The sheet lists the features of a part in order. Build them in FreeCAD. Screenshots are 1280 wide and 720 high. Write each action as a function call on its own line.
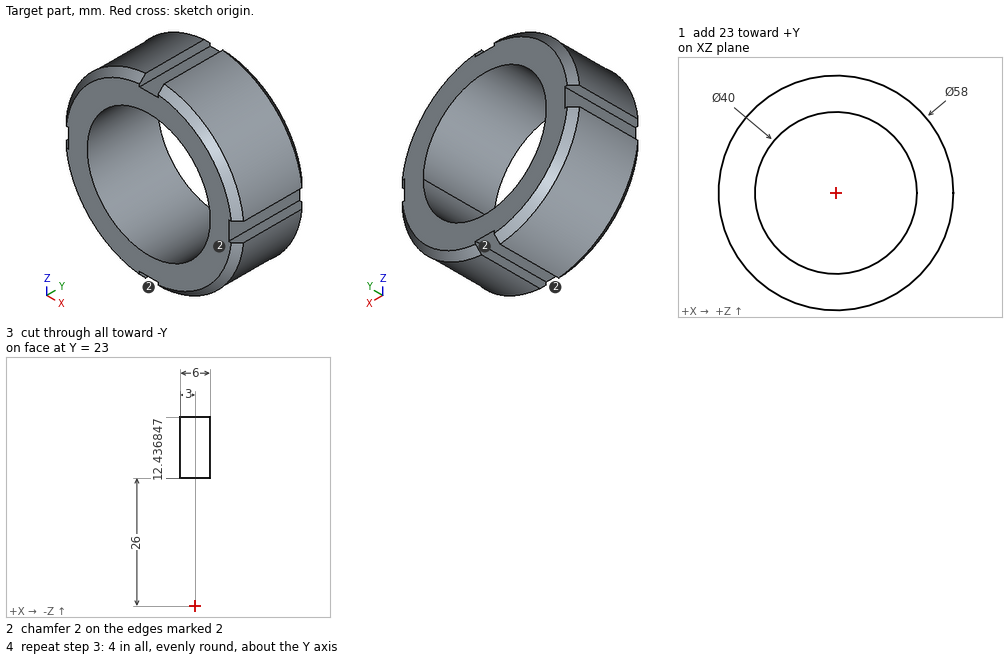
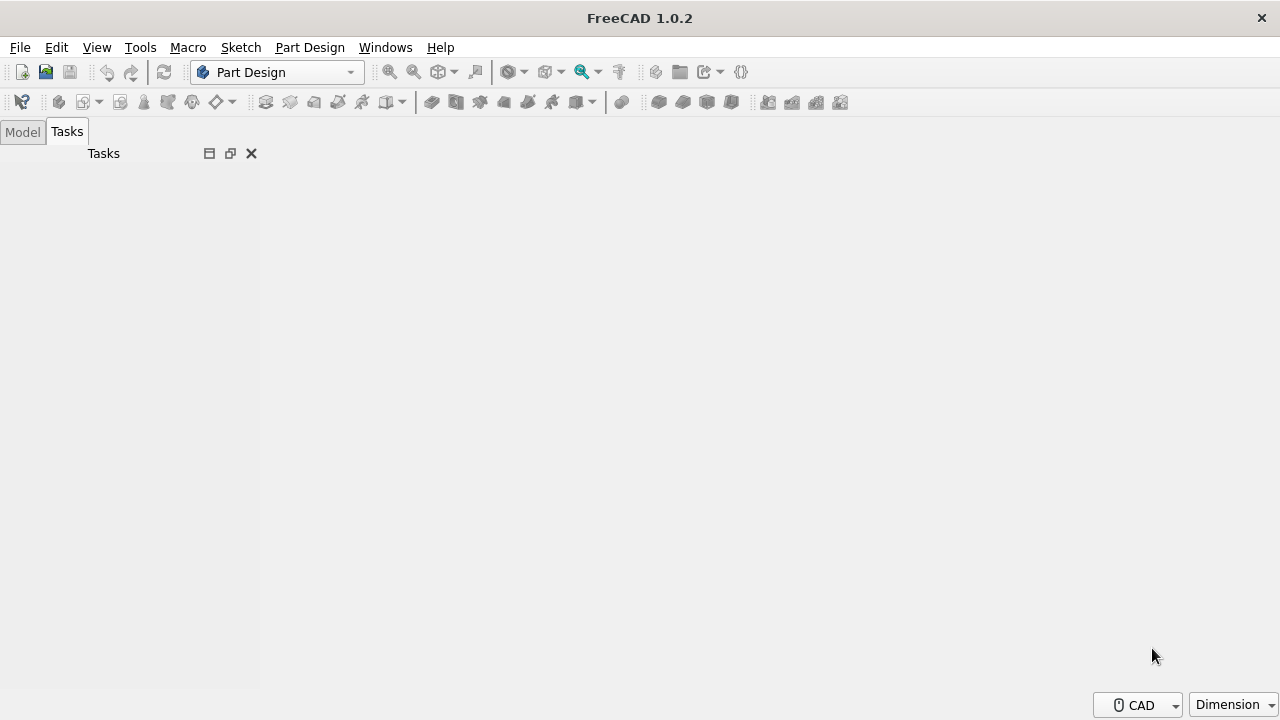
click(22, 72)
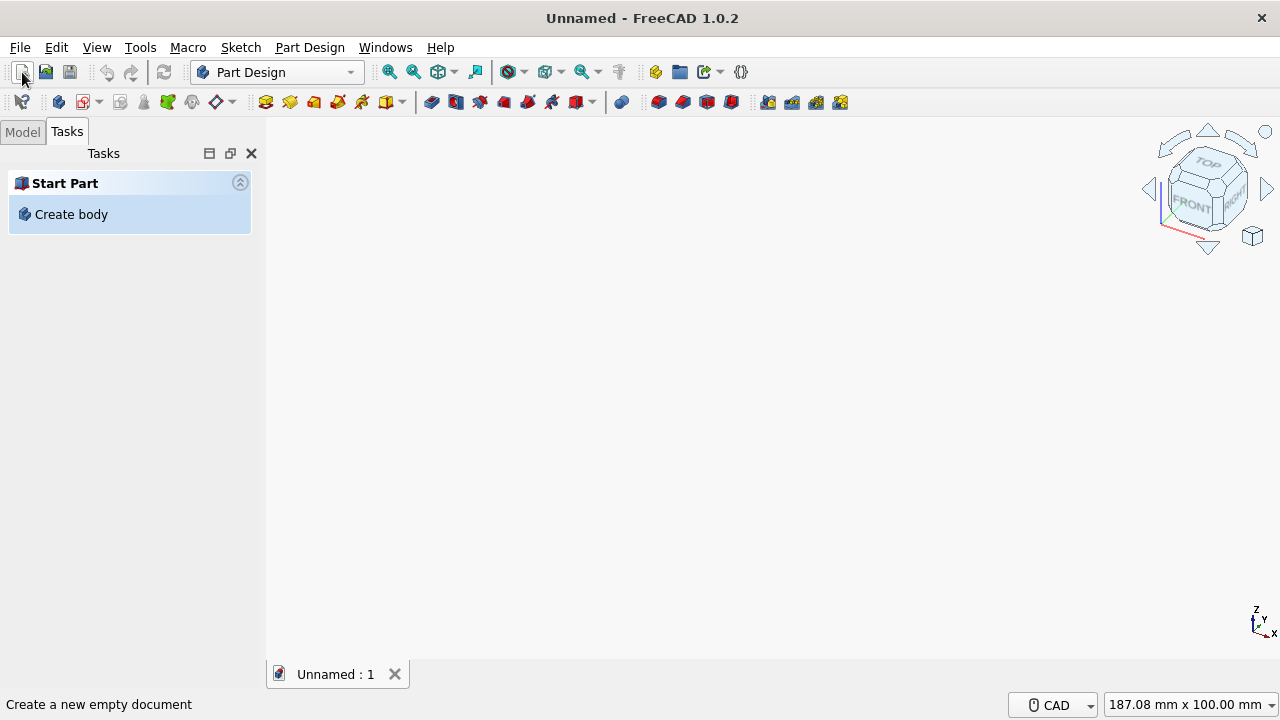
click(84, 102)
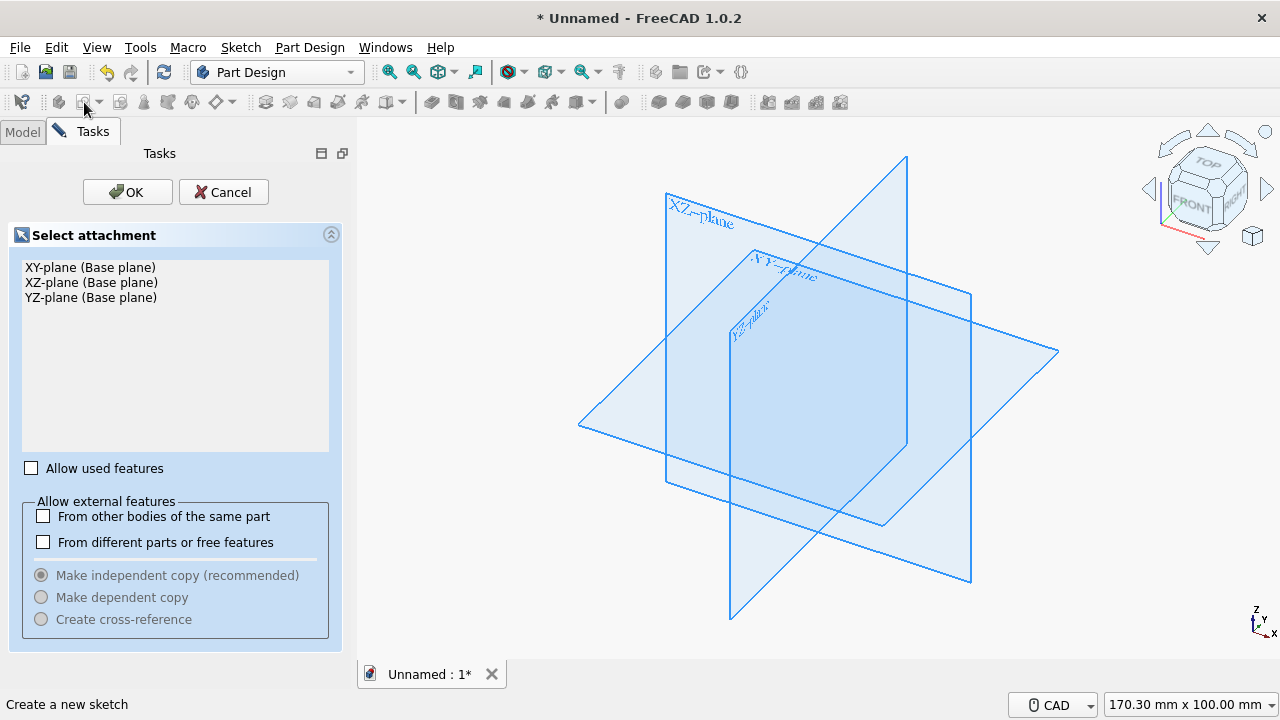
click(82, 282)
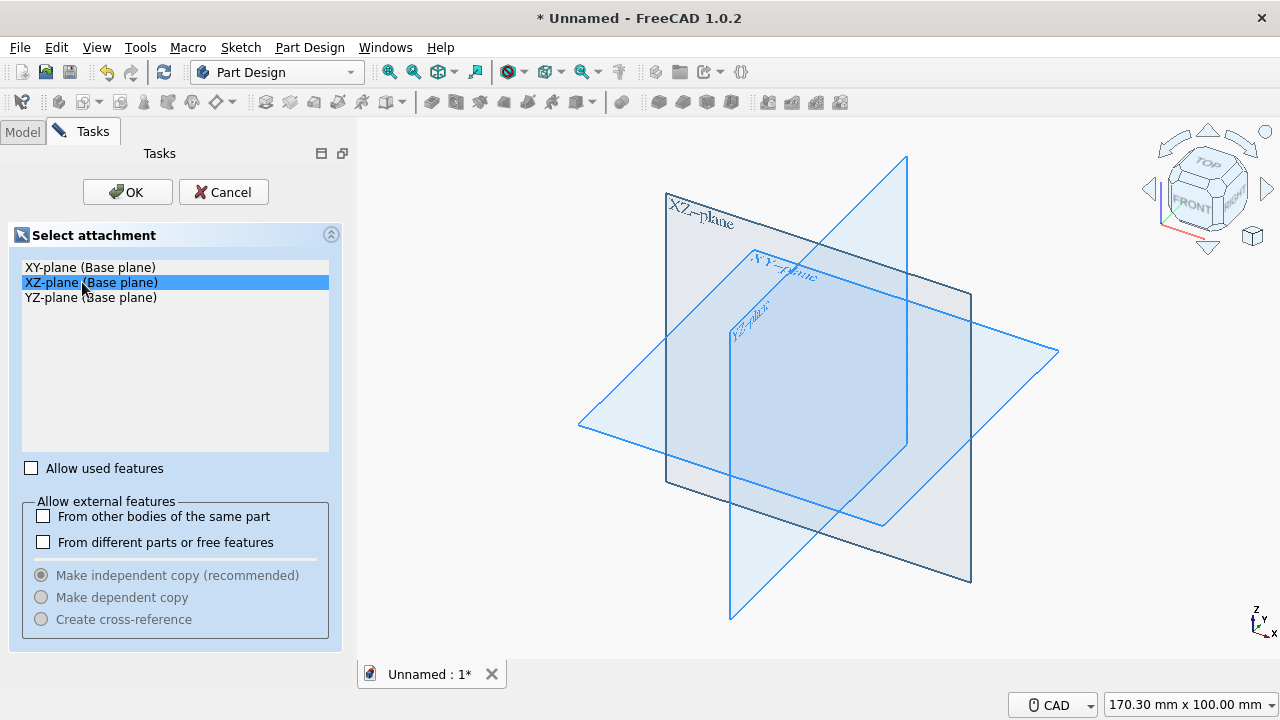
click(128, 192)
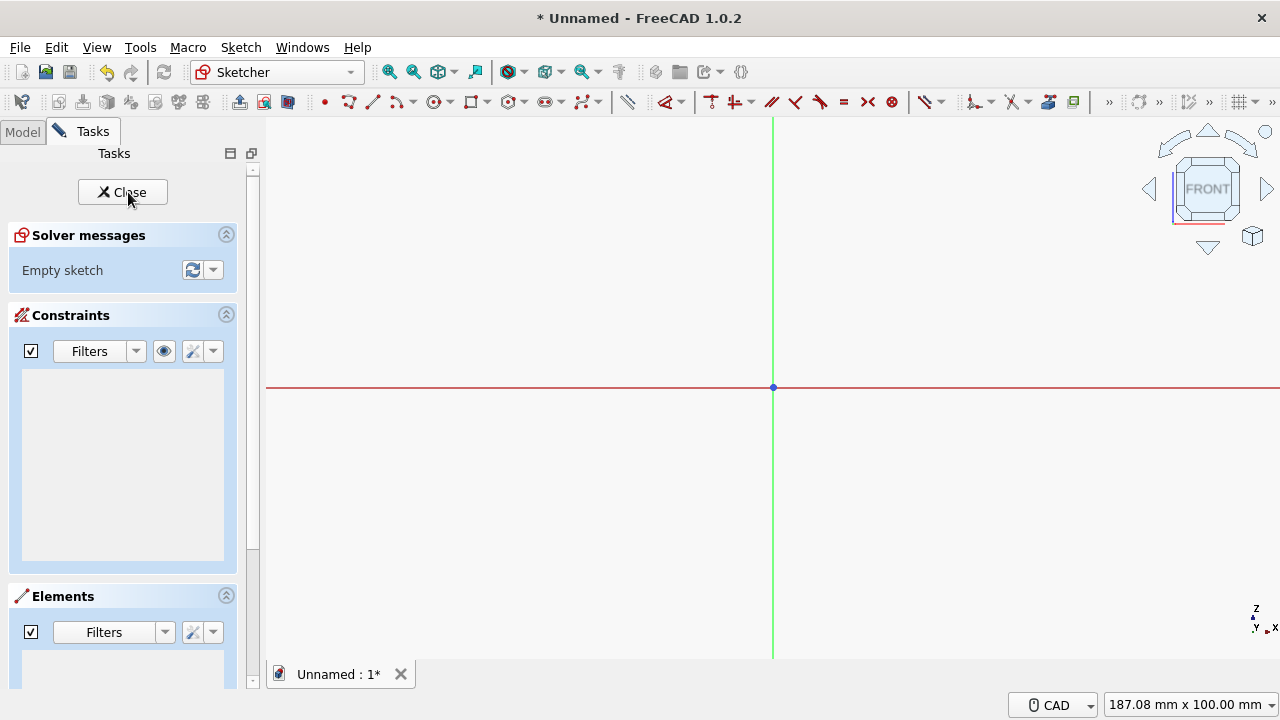
click(434, 102)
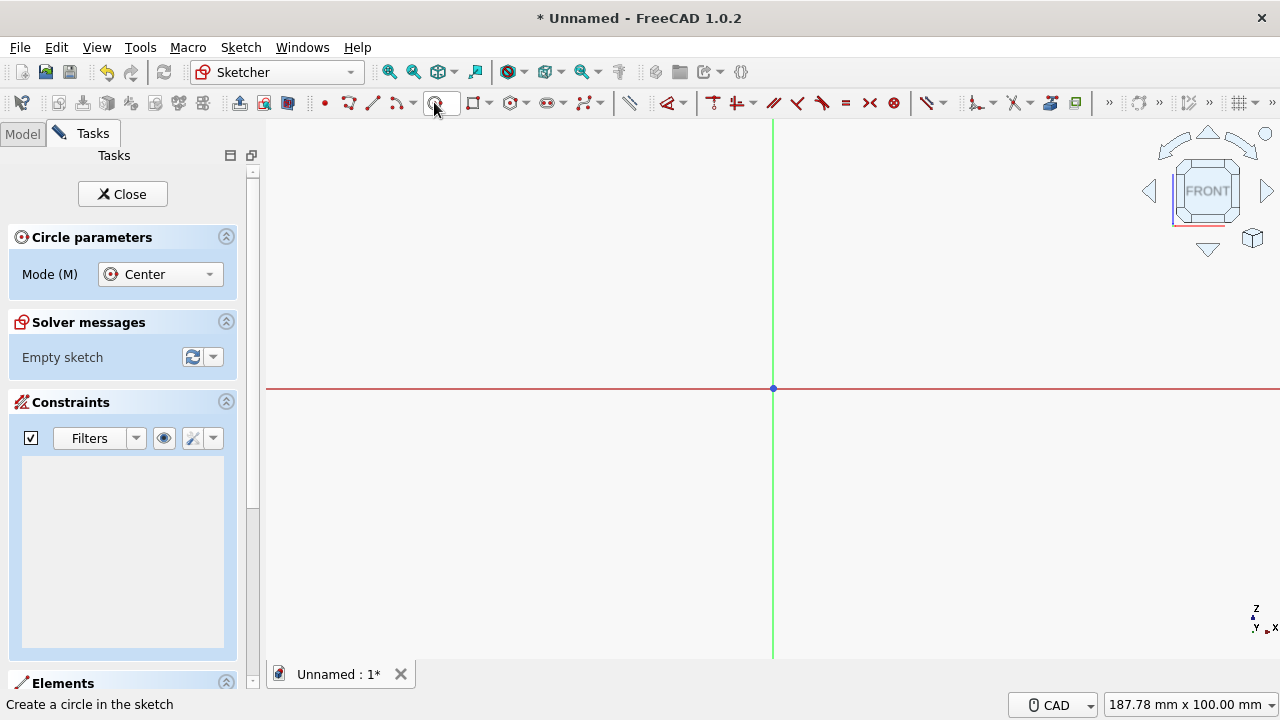
click(773, 389)
click(884, 278)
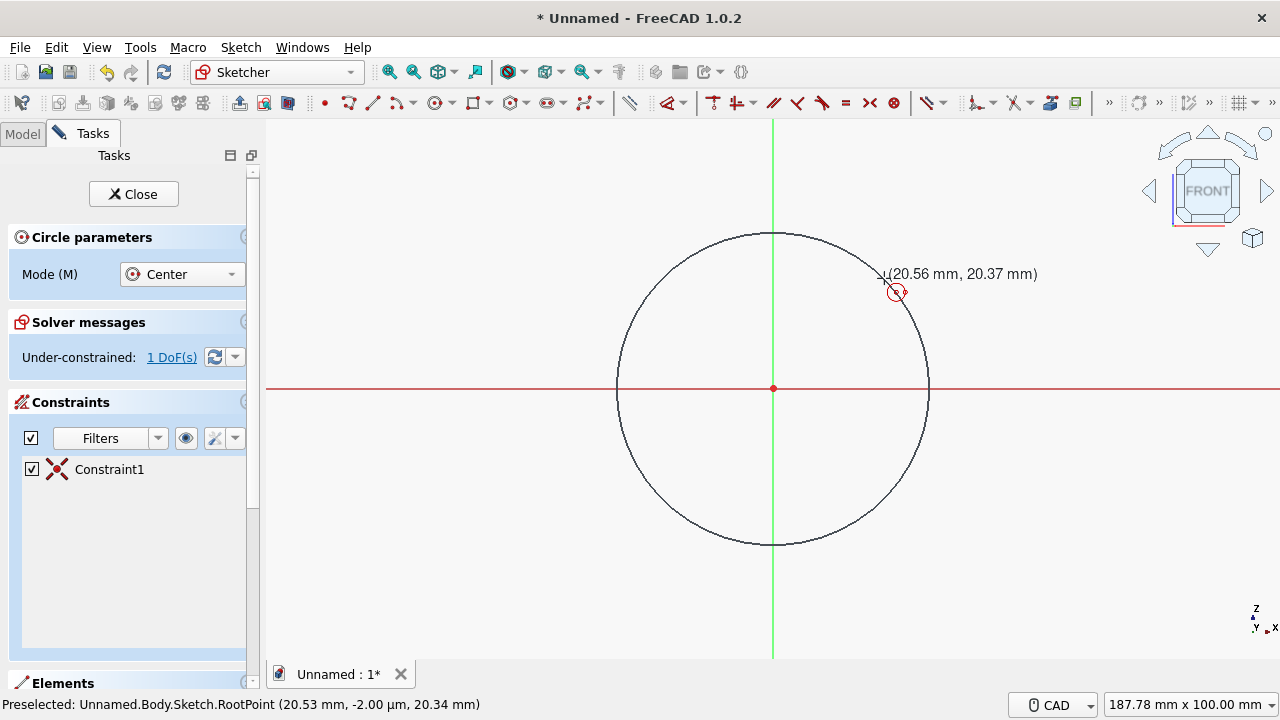
click(773, 389)
click(849, 313)
key(Escape)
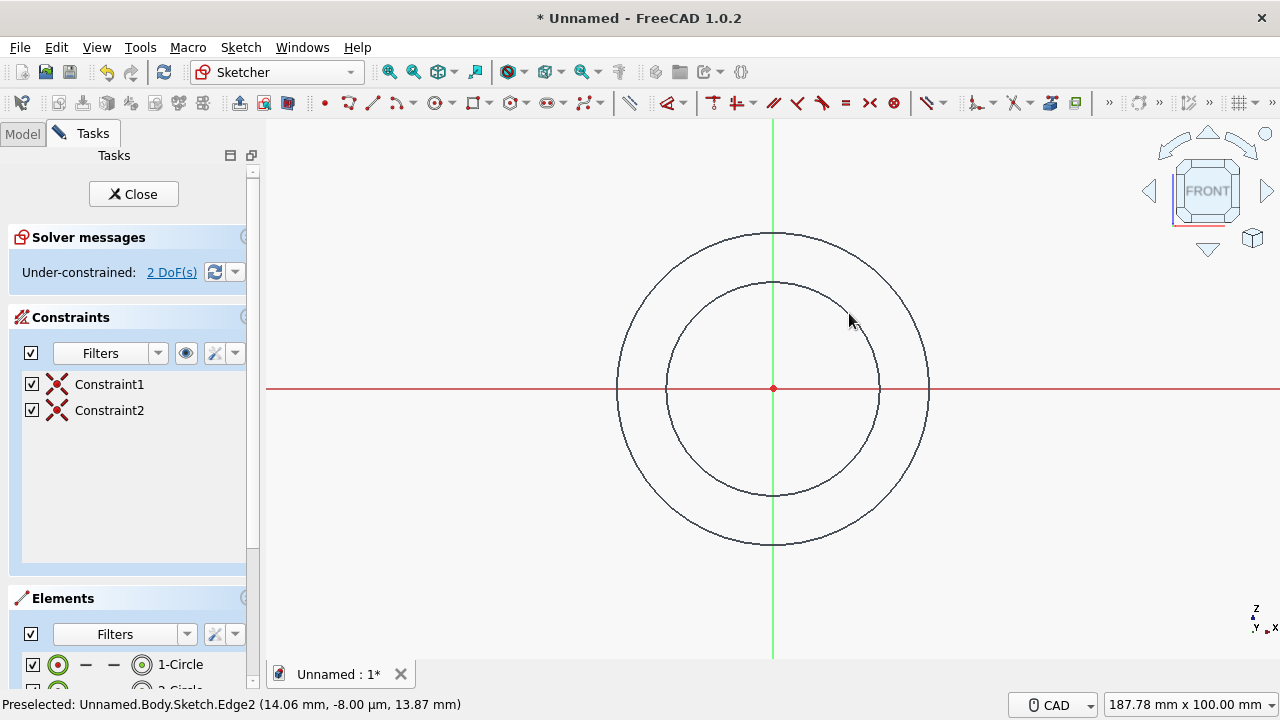
click(668, 104)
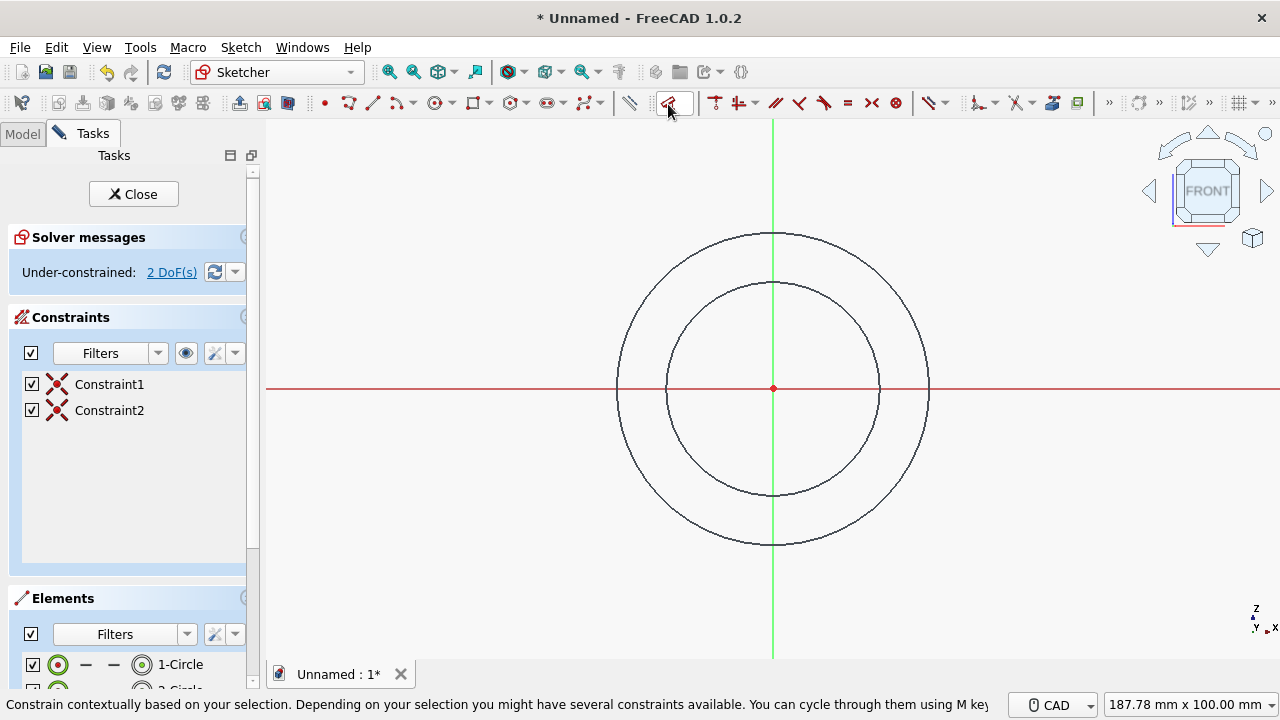
click(883, 278)
click(906, 255)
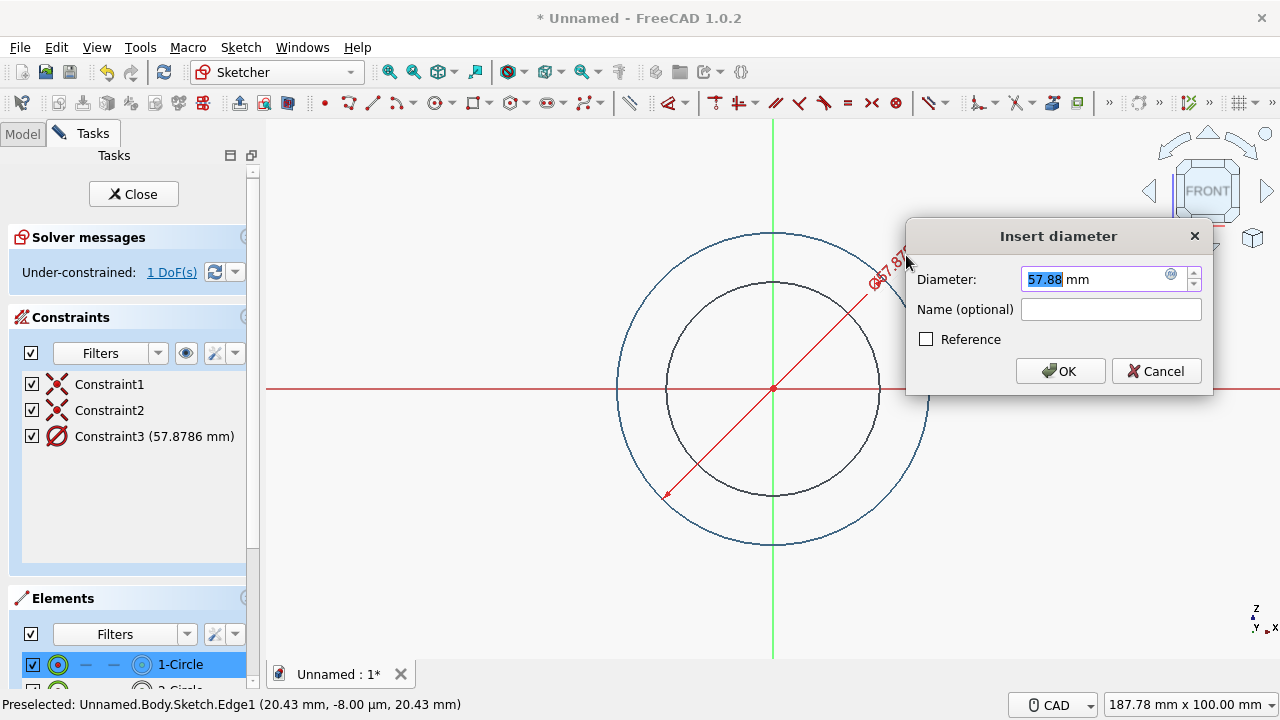
text(58)
key(Return)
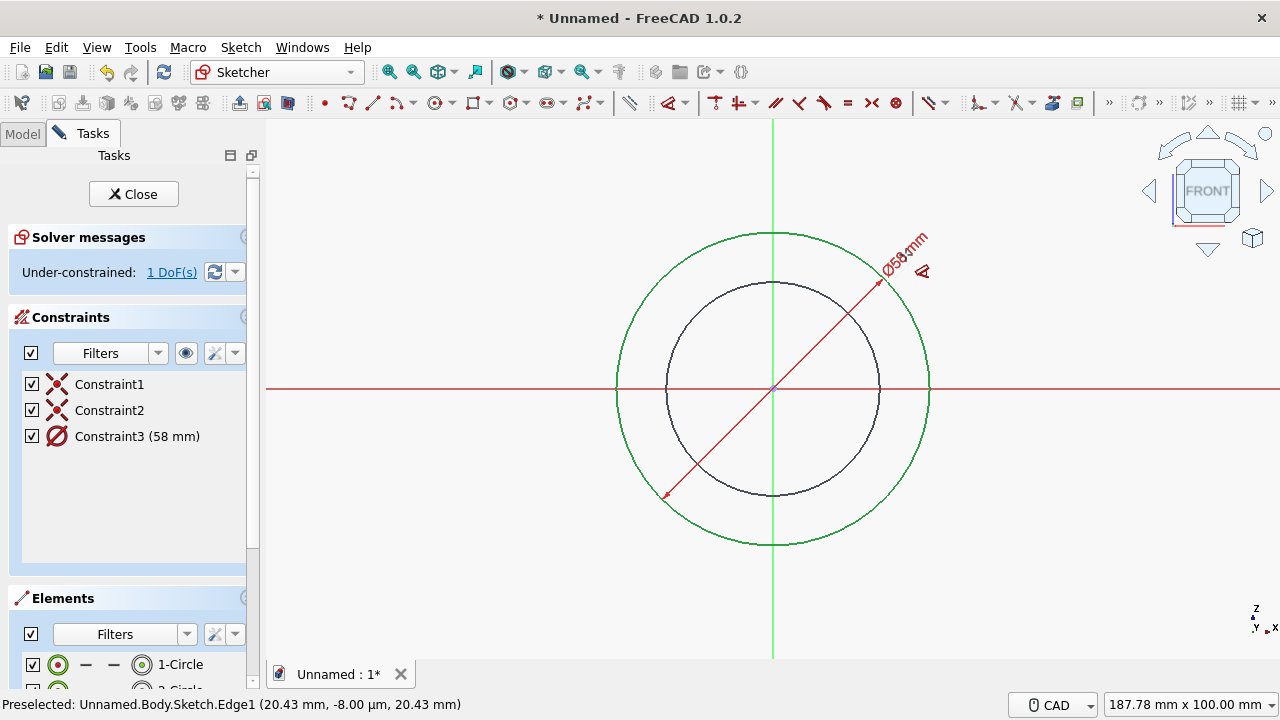
click(848, 313)
click(870, 290)